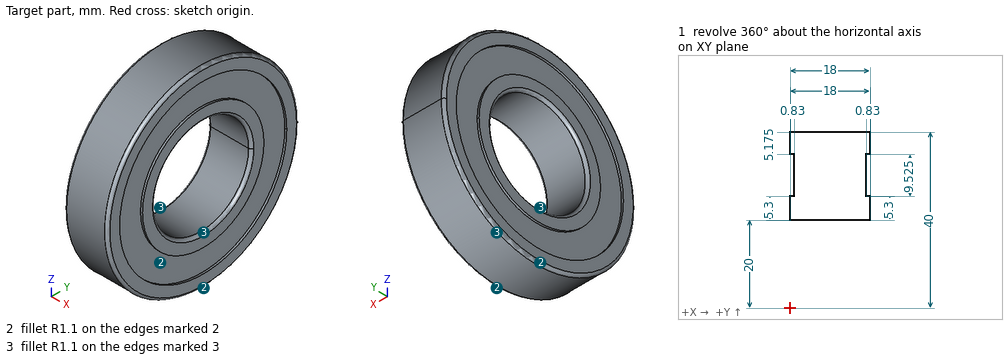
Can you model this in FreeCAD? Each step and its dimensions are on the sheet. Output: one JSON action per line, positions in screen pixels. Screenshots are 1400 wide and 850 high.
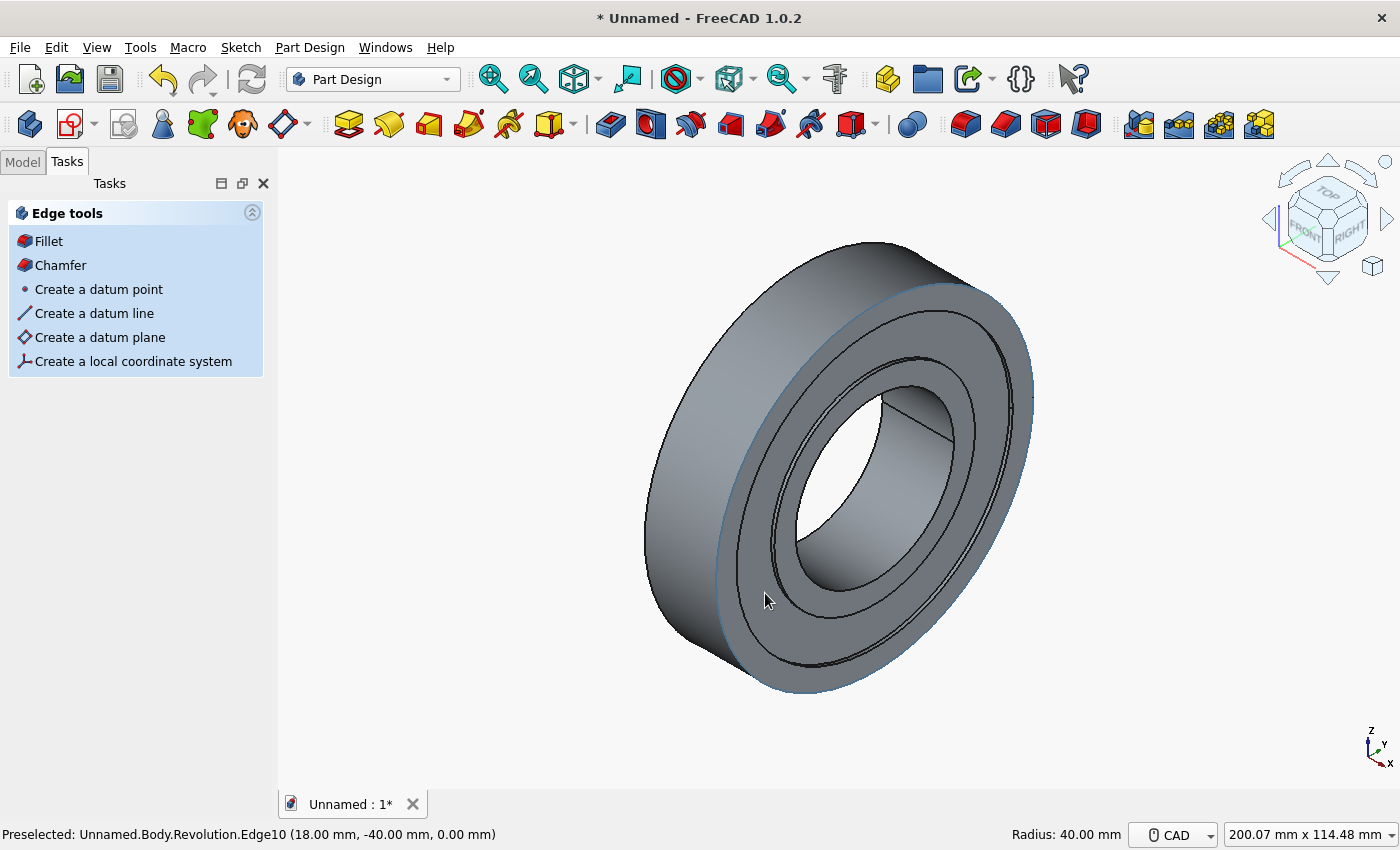
{"action": "key", "text": "2"}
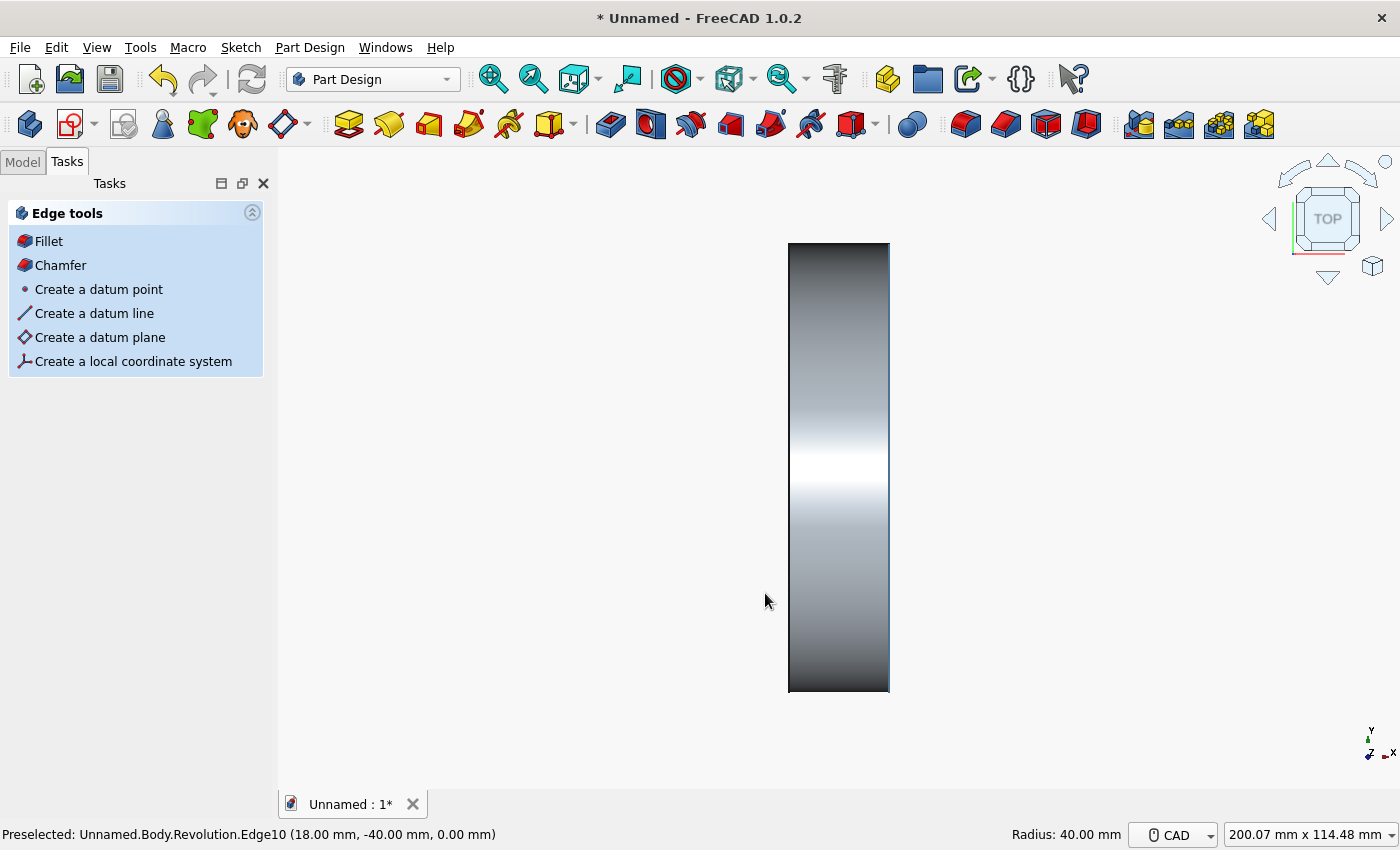
{"action": "left_click", "coordinate": [789, 648], "text": "ctrl"}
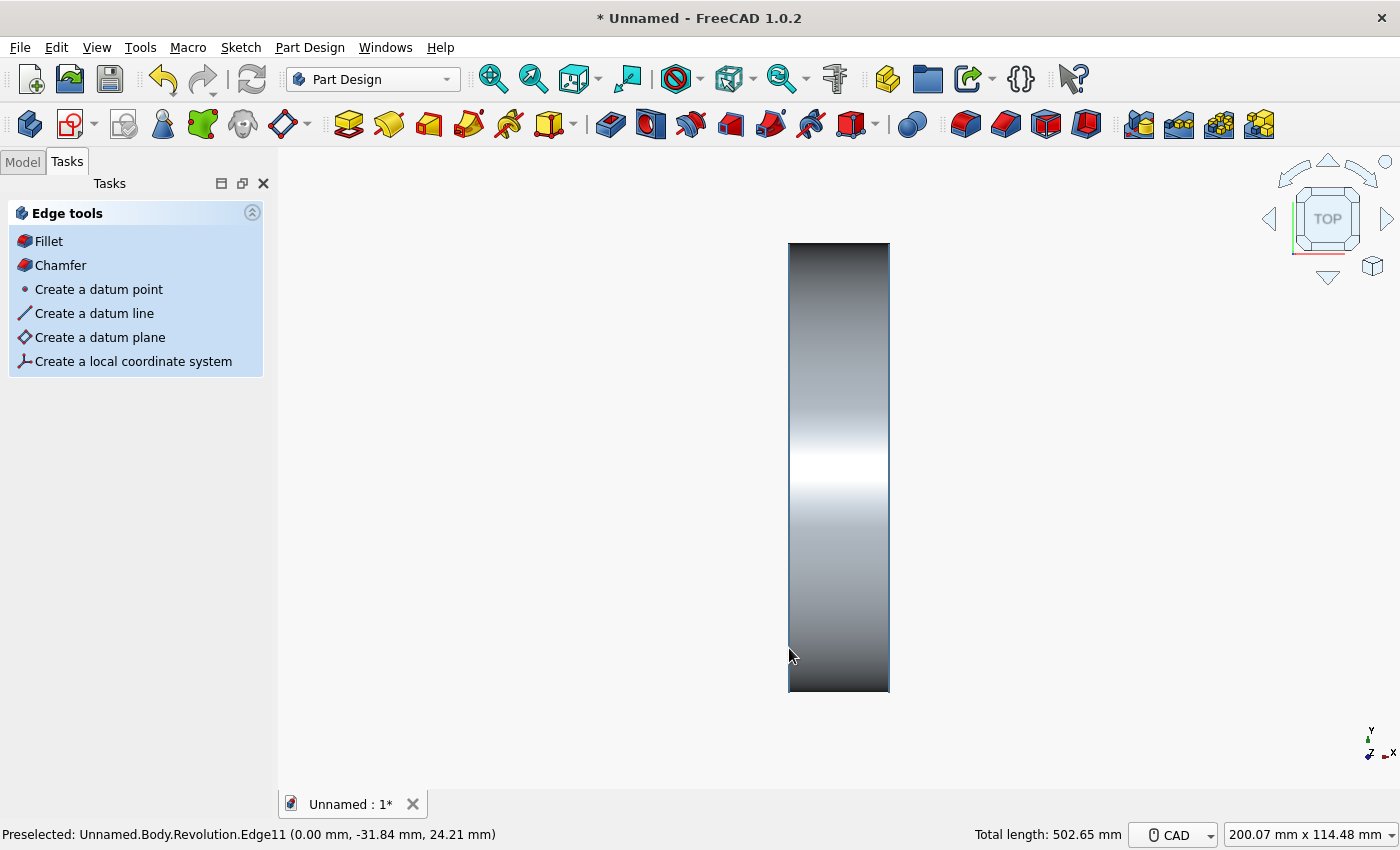
{"action": "left_click", "coordinate": [966, 124]}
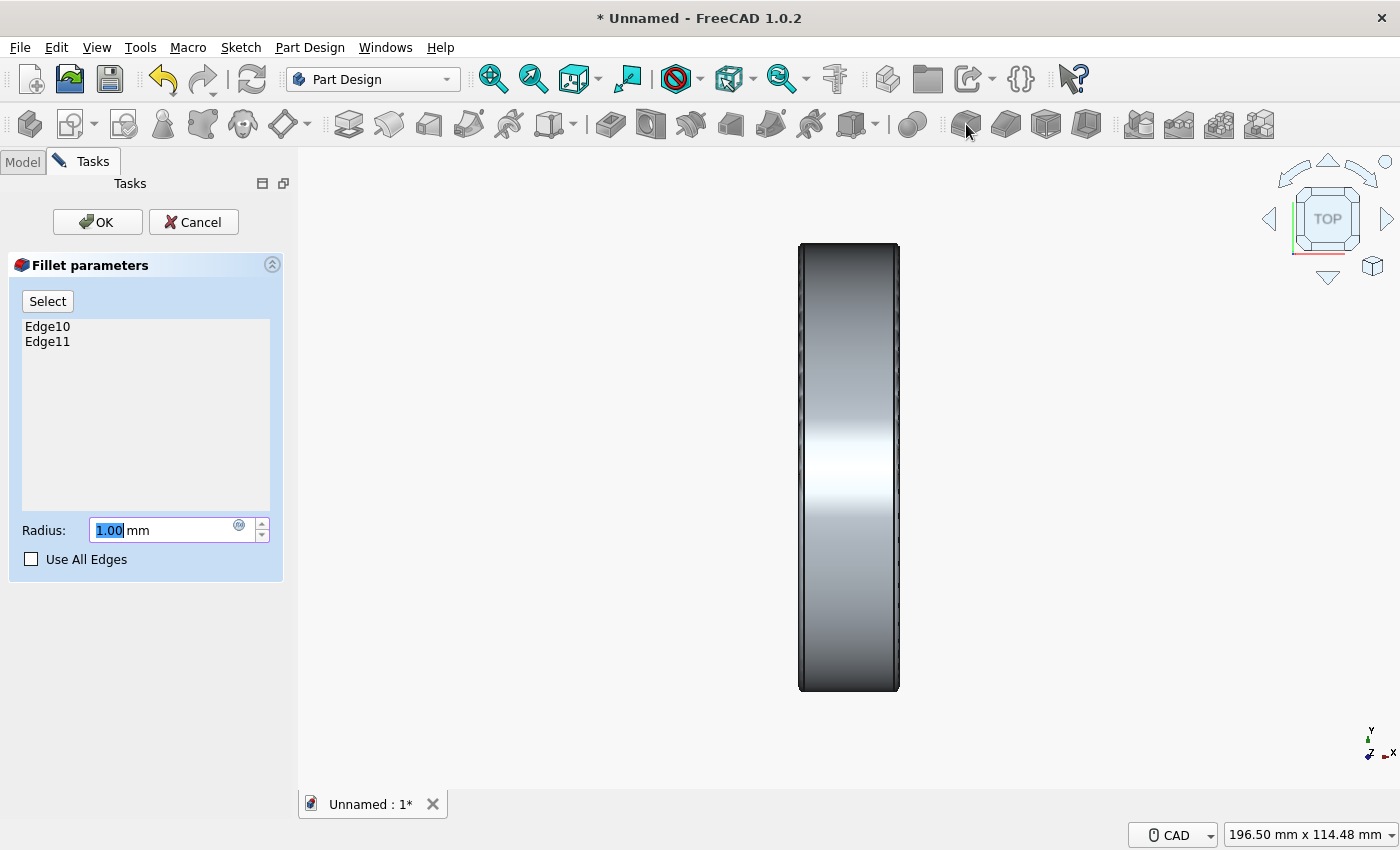
{"action": "type", "text": "1.1"}
{"action": "key", "text": "Tab"}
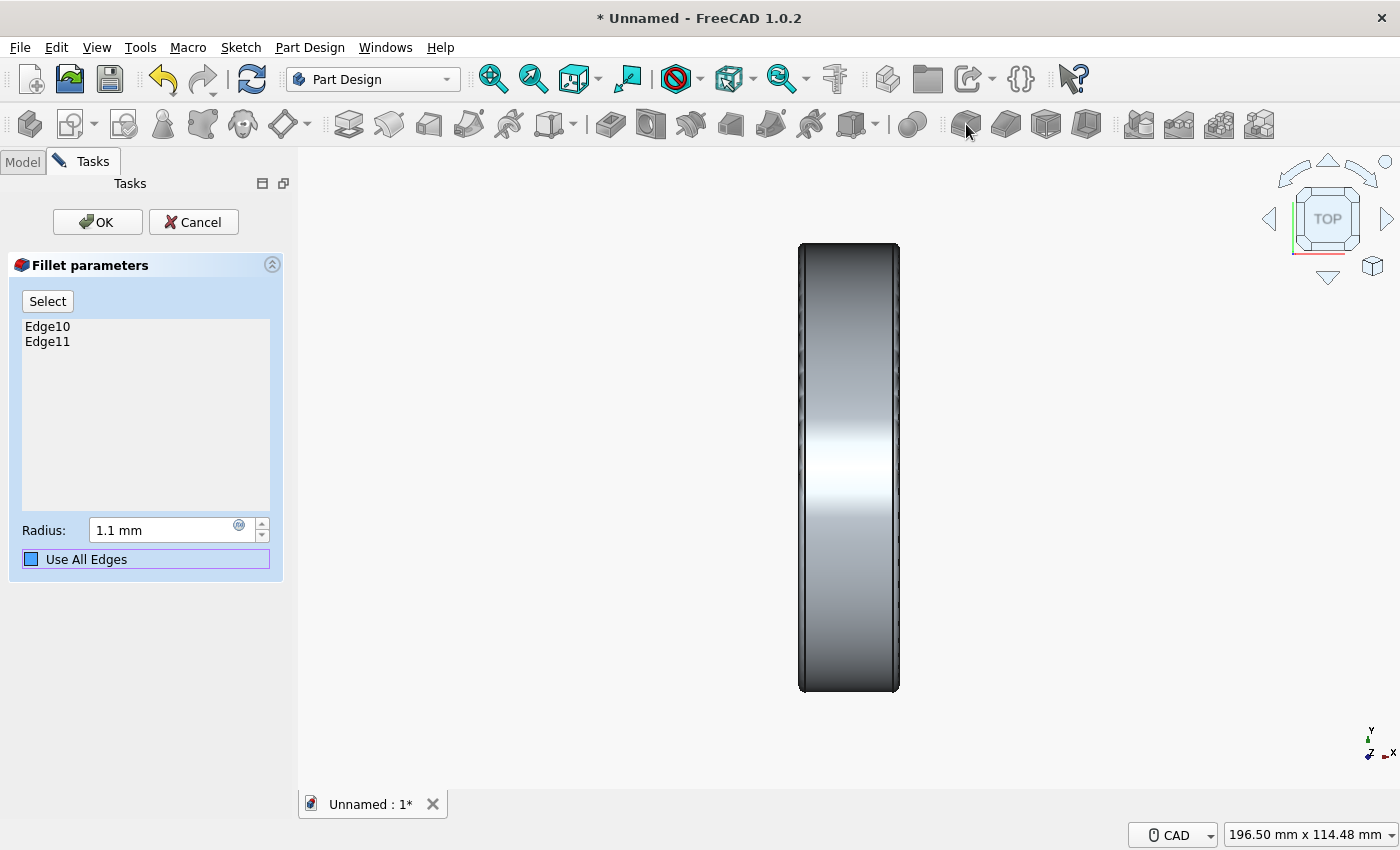
{"action": "left_click", "coordinate": [98, 222]}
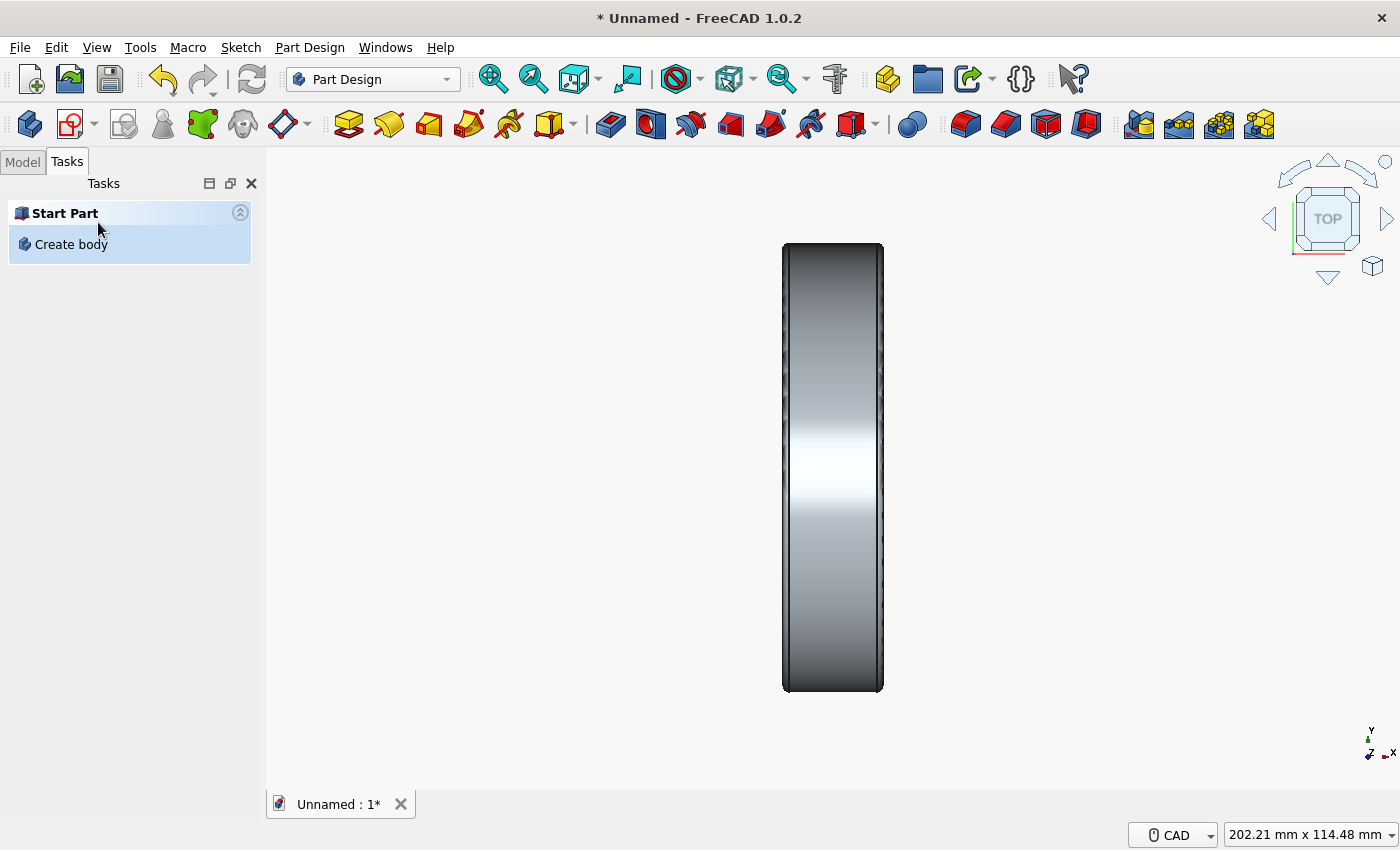
{"action": "key", "text": "0"}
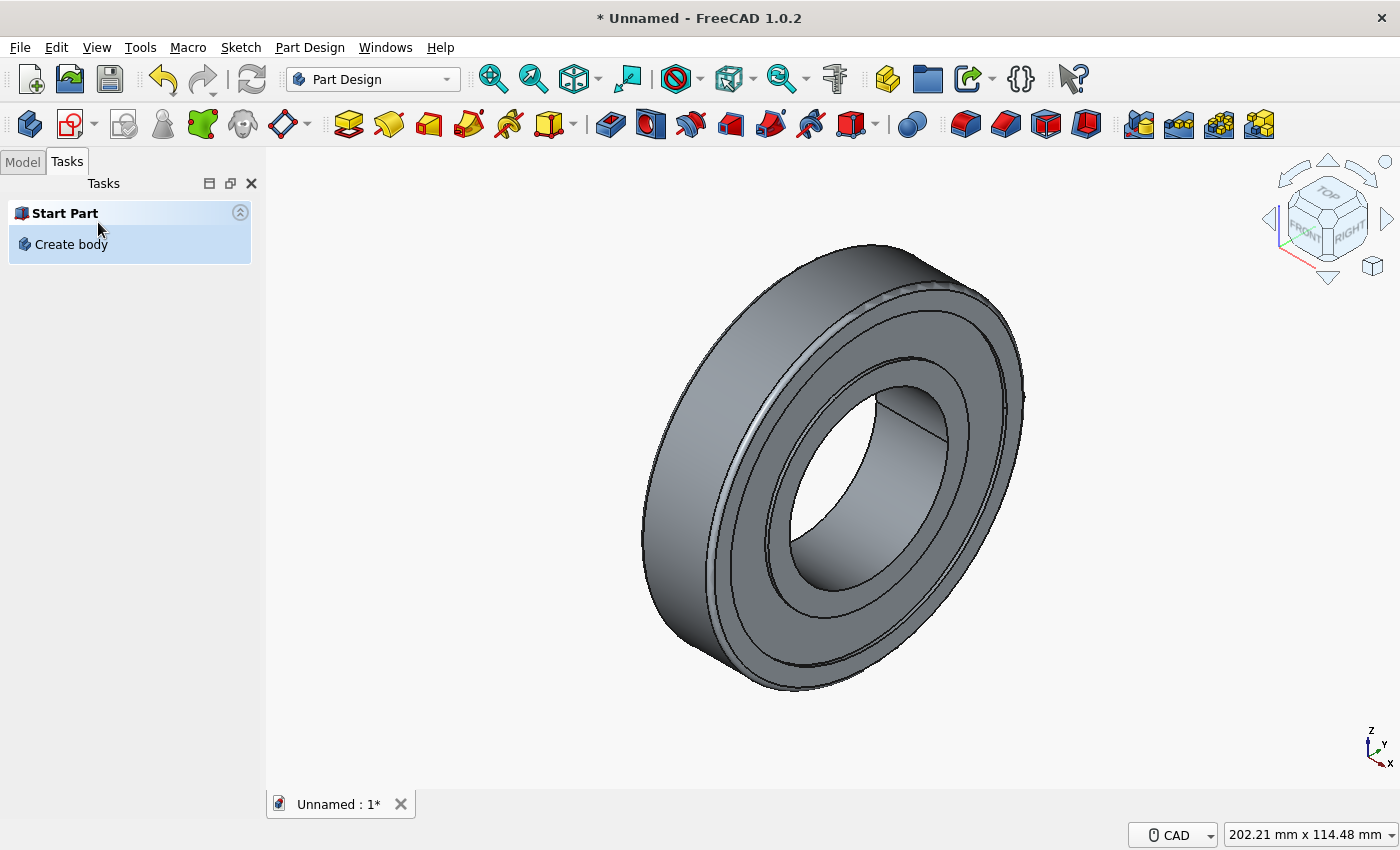
{"action": "left_click", "coordinate": [844, 589]}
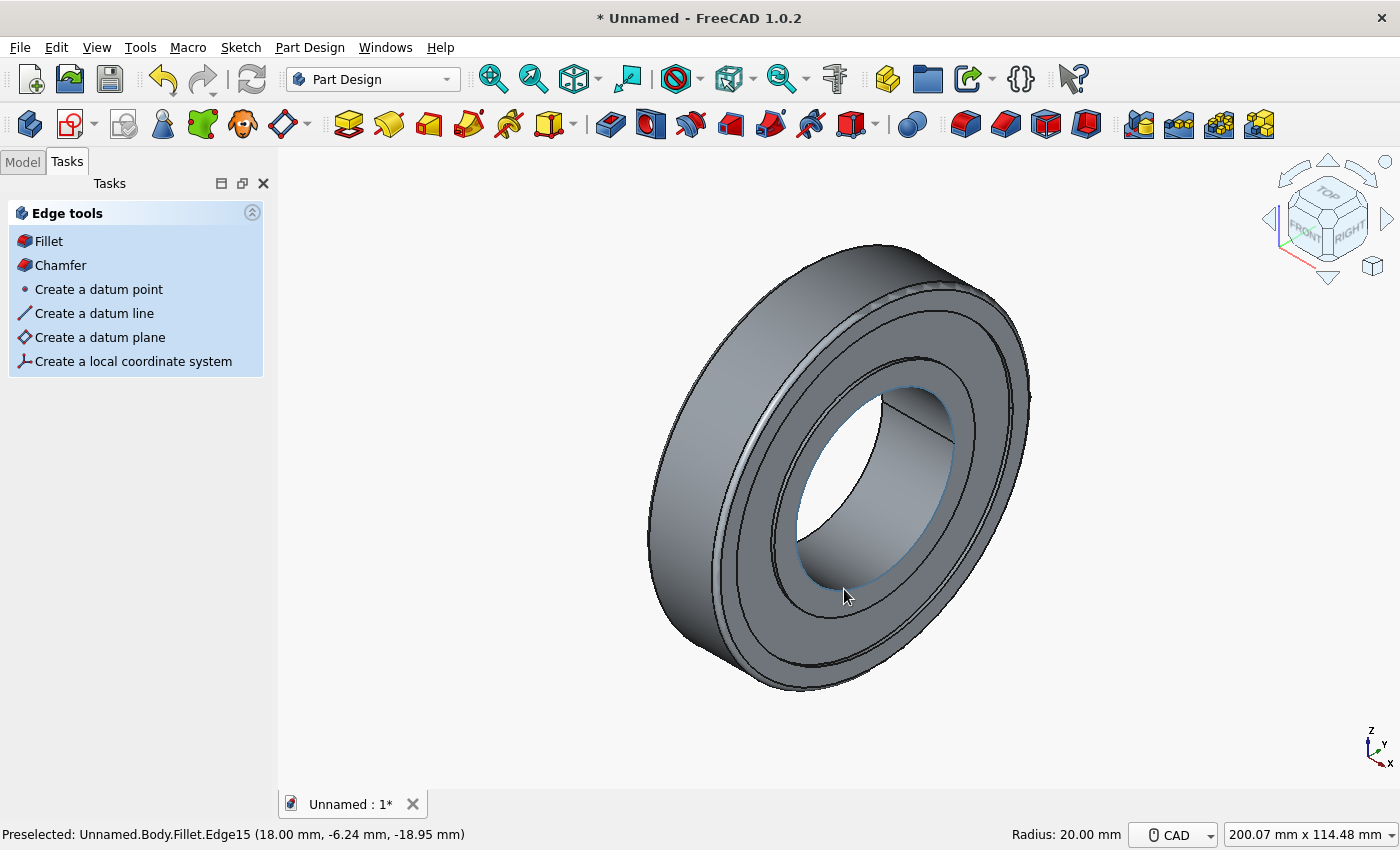
{"action": "key", "text": "2"}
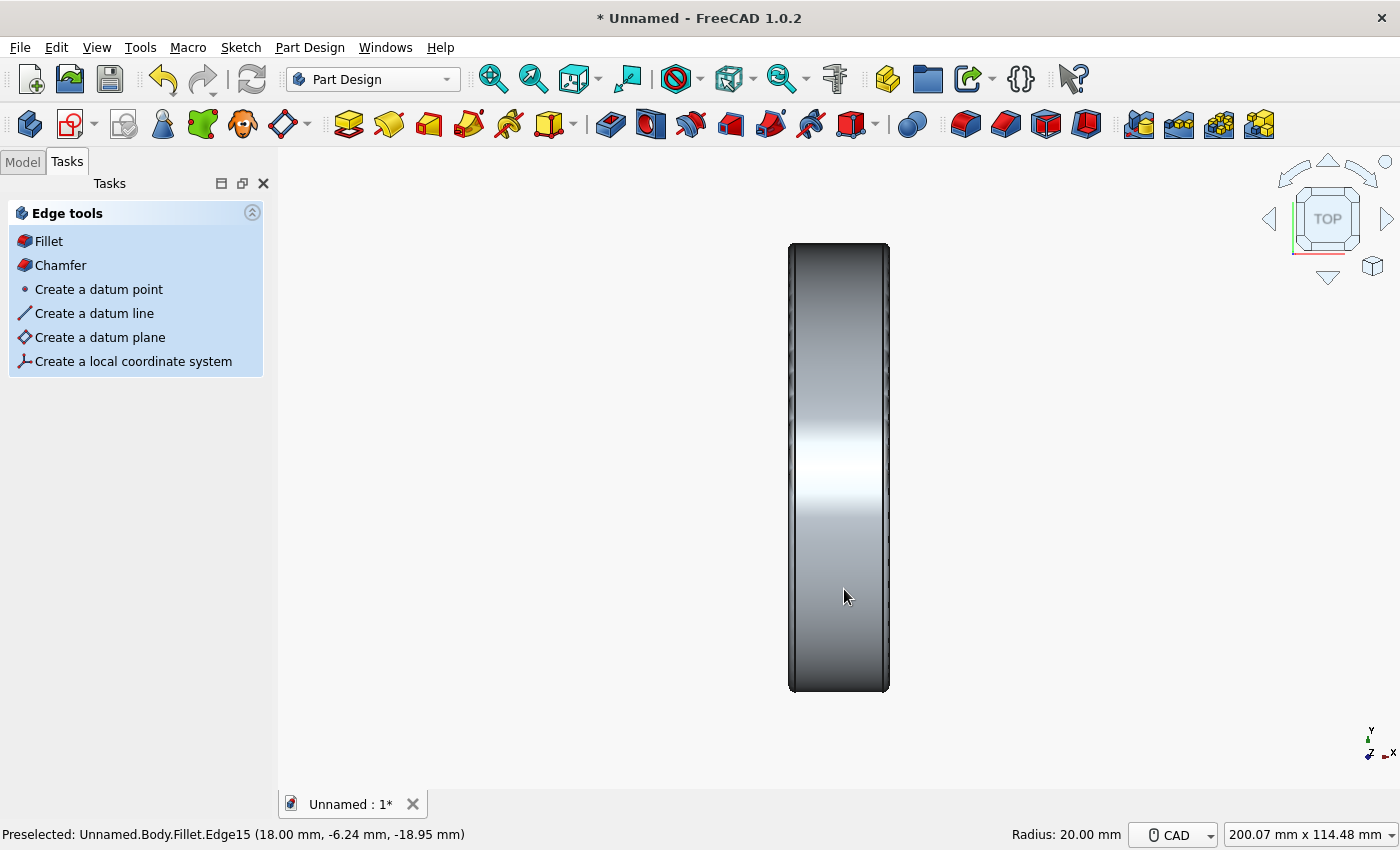
{"action": "key", "text": "1"}